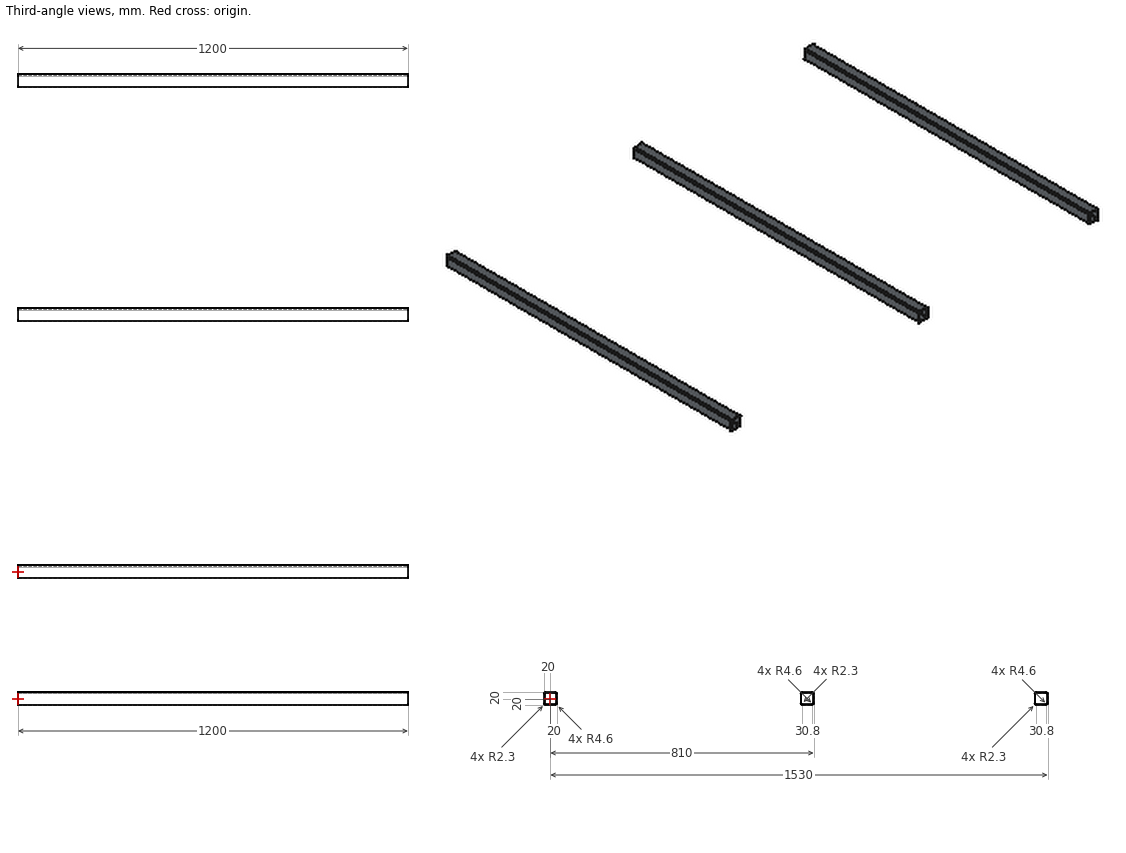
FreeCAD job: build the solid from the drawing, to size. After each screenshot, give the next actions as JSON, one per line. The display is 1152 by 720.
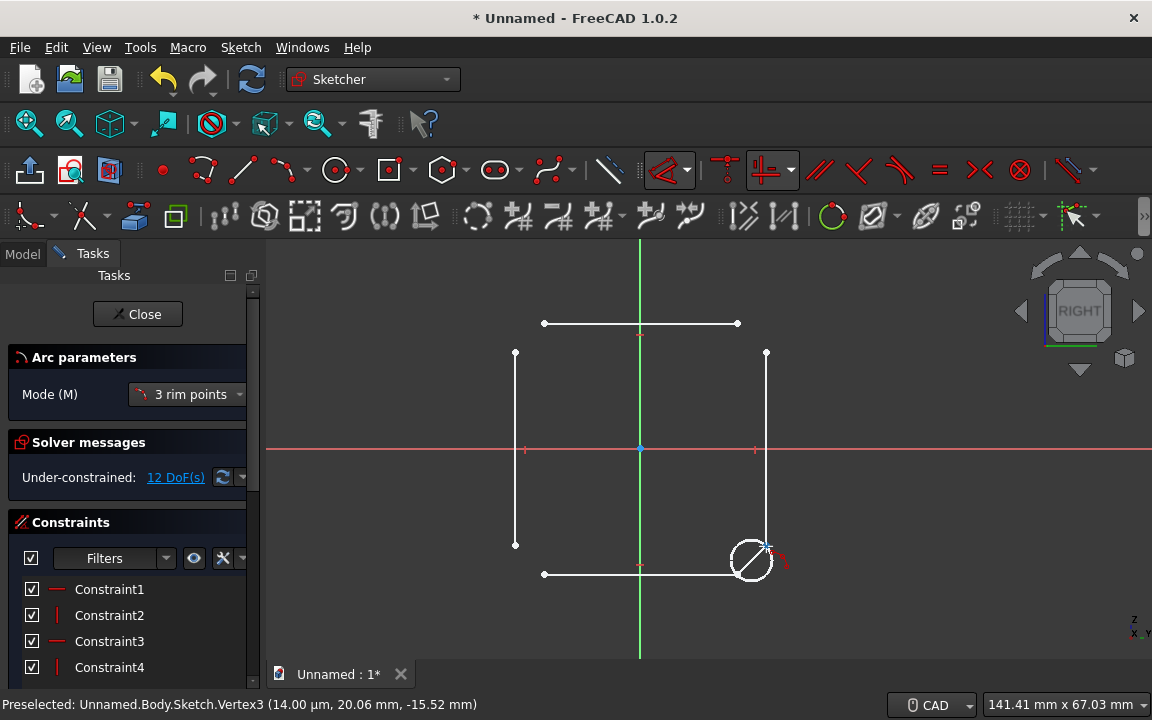
{"action": "scroll", "coordinate": [757, 566], "scroll_direction": "up", "scroll_amount": 4}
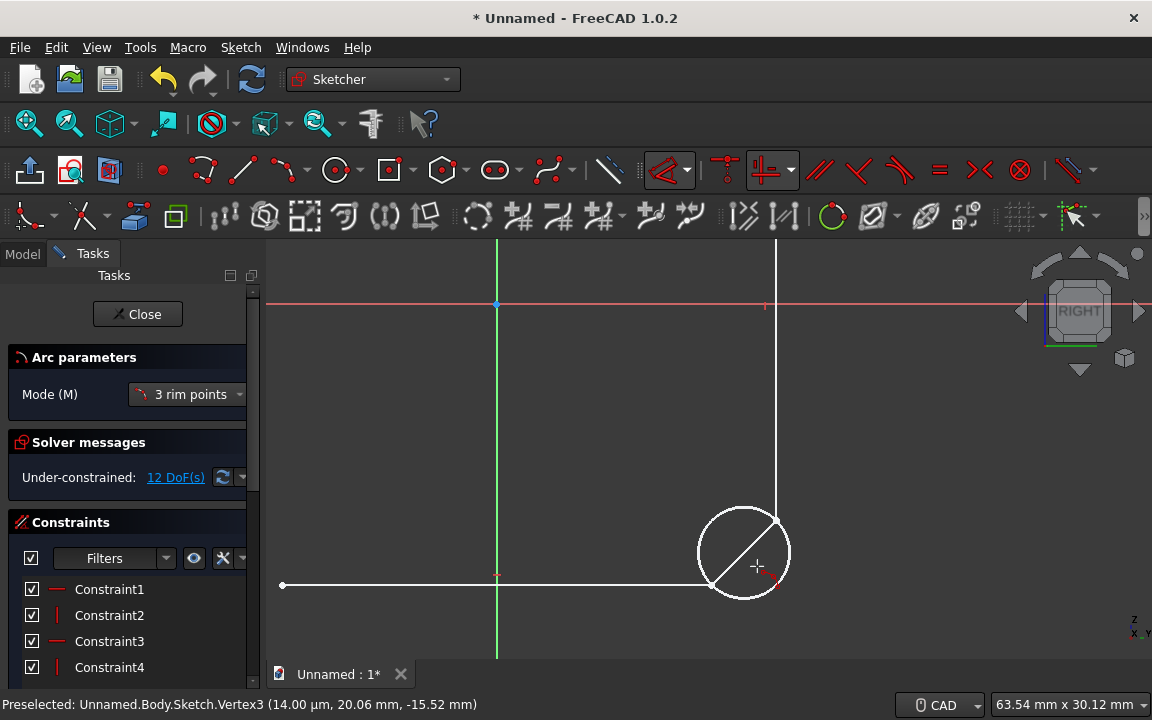
{"action": "left_click", "coordinate": [757, 564]}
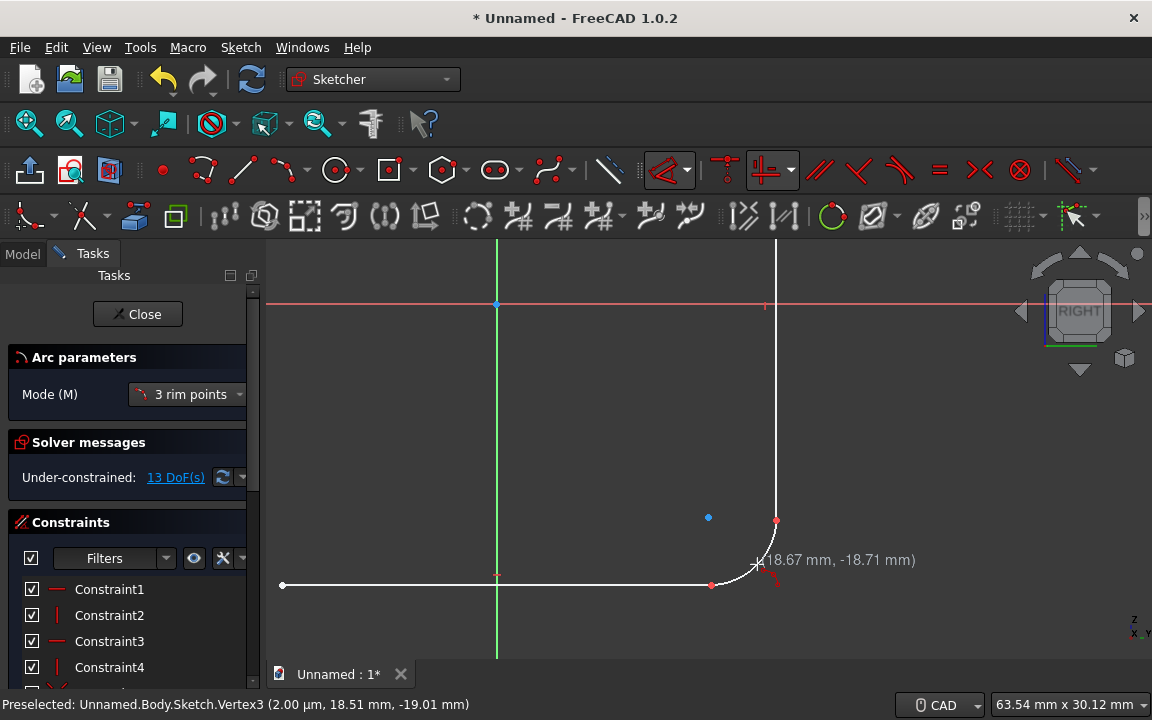
{"action": "scroll", "coordinate": [758, 567], "scroll_direction": "down", "scroll_amount": 4}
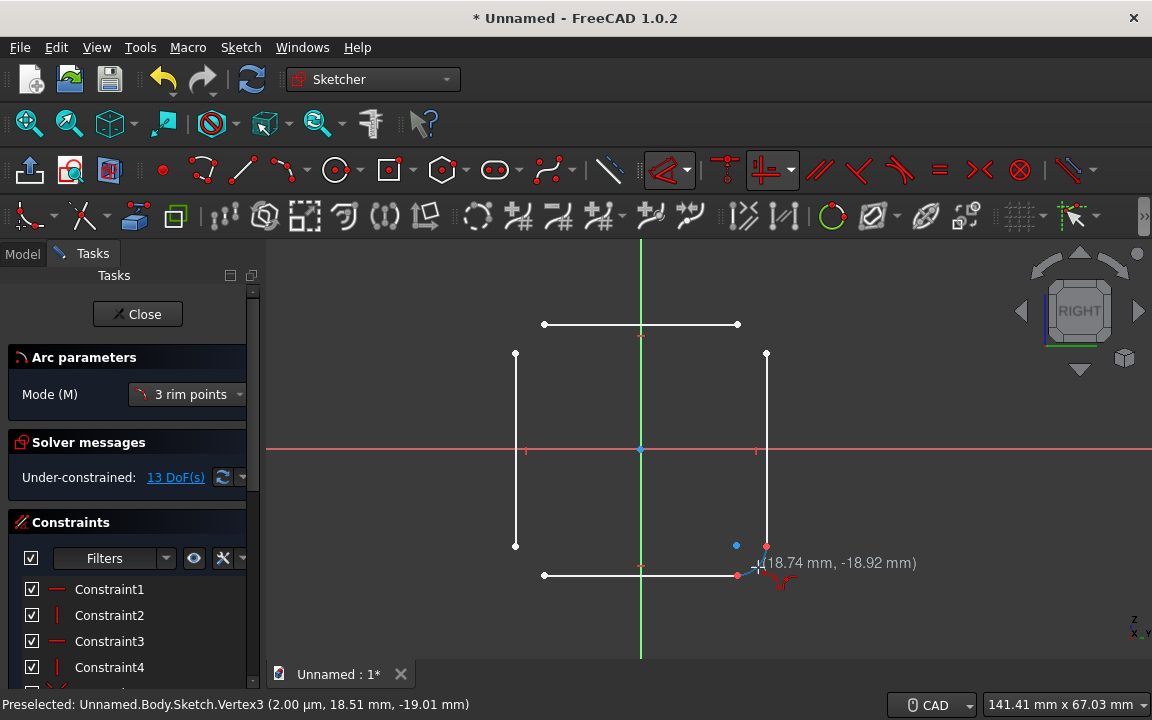
{"action": "left_click", "coordinate": [767, 354]}
{"action": "left_click", "coordinate": [738, 325]}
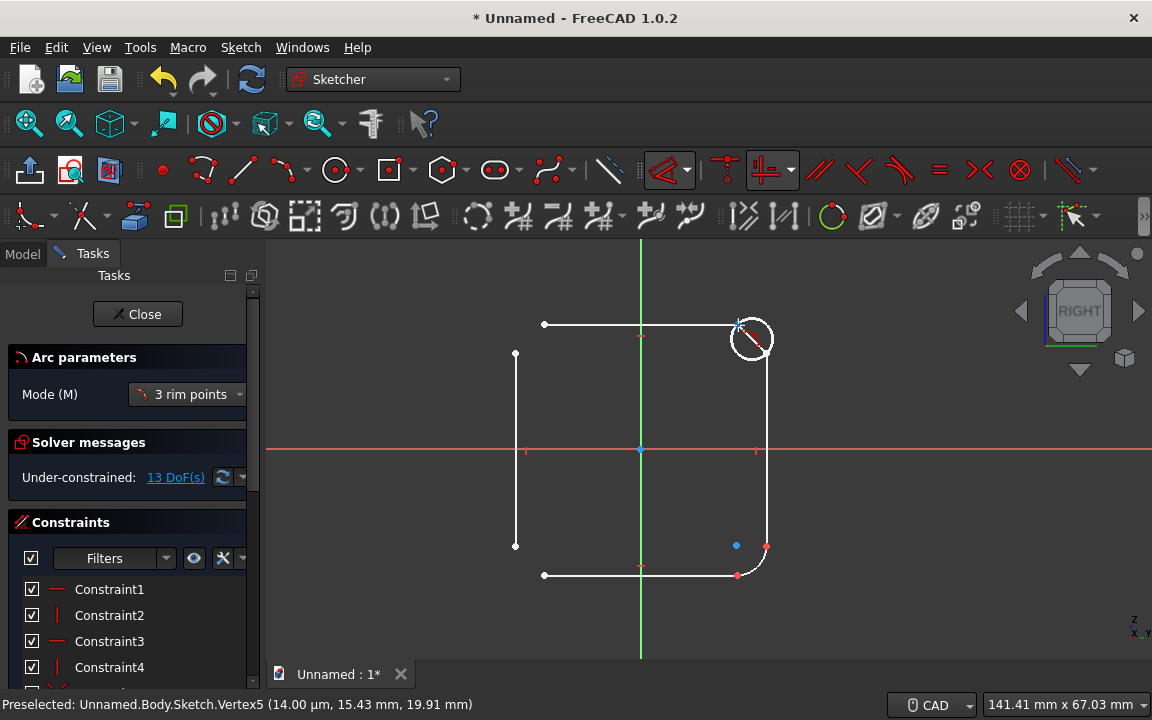
{"action": "scroll", "coordinate": [758, 332], "scroll_direction": "up", "scroll_amount": 4}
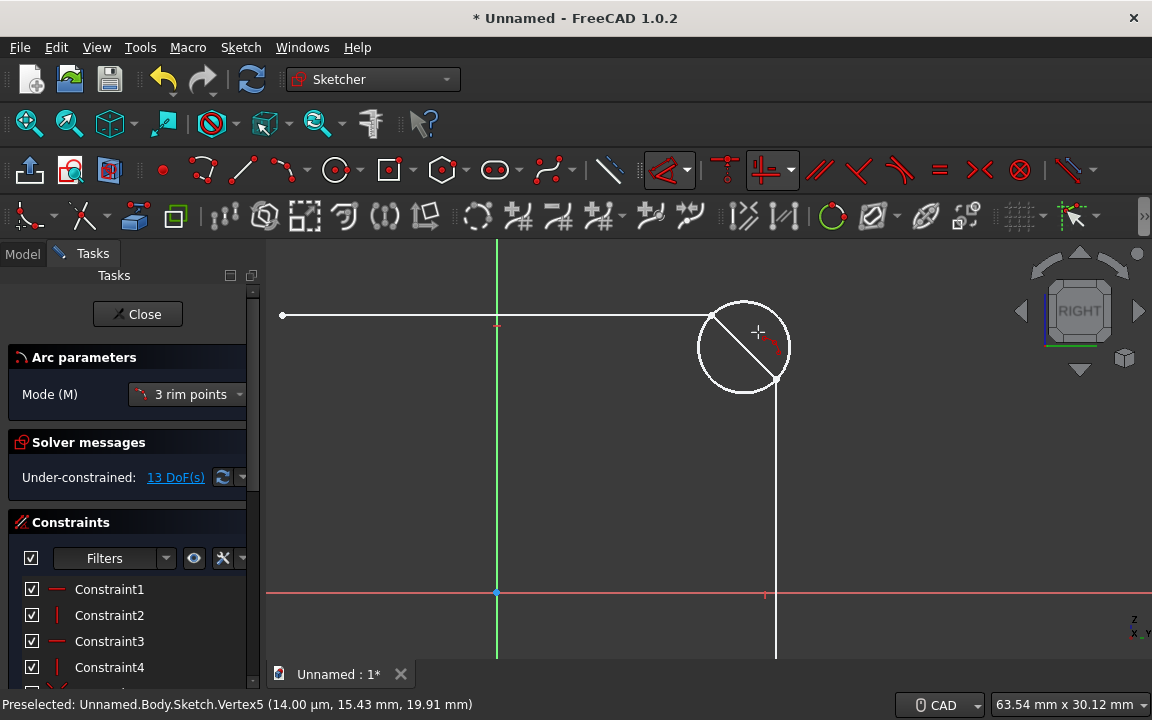
{"action": "left_click", "coordinate": [757, 333]}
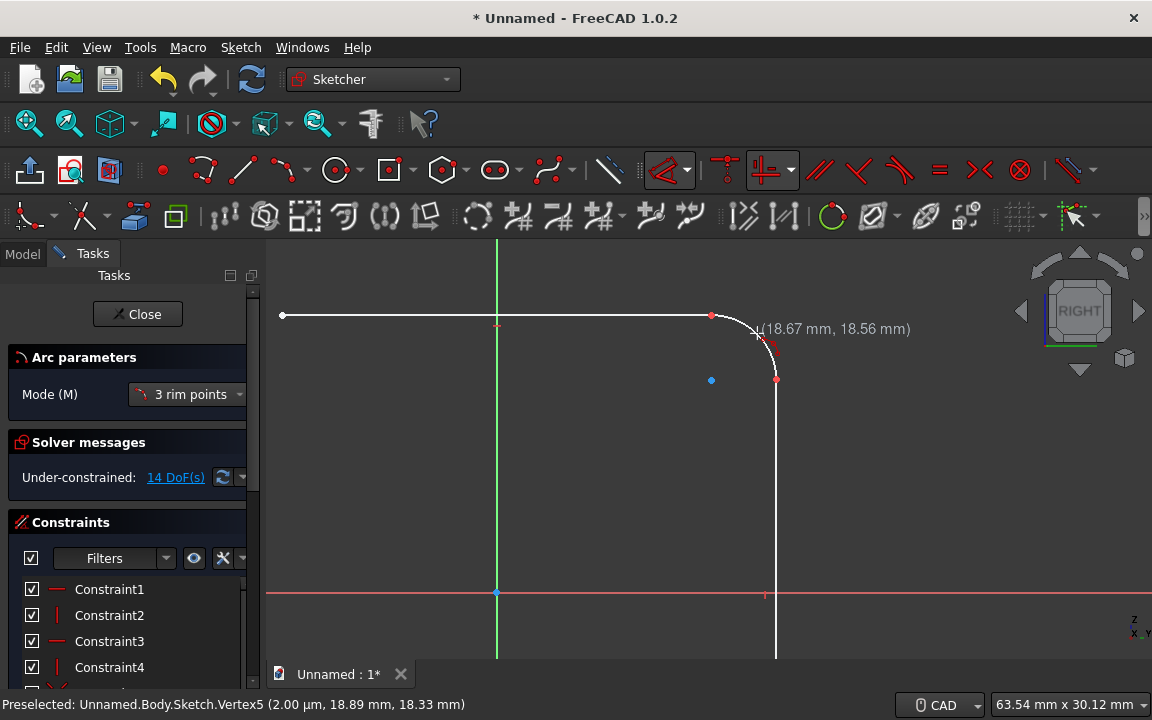
{"action": "scroll", "coordinate": [758, 332], "scroll_direction": "down", "scroll_amount": 4}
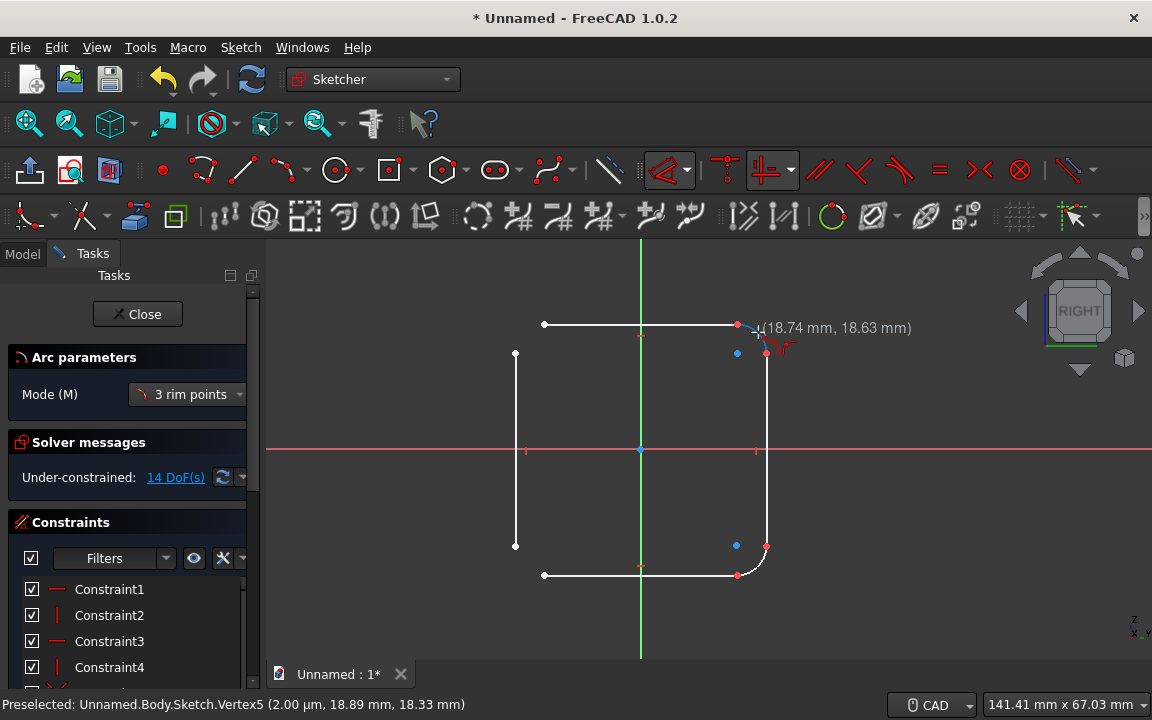
{"action": "left_click", "coordinate": [545, 325]}
{"action": "left_click", "coordinate": [516, 354]}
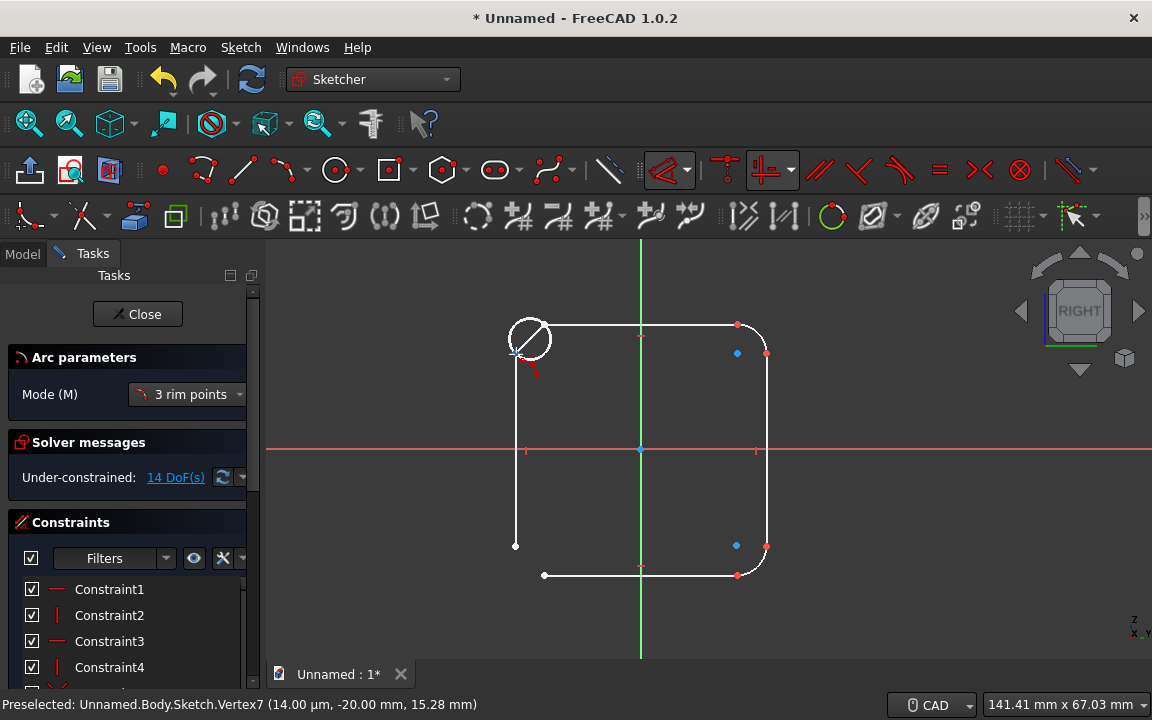
{"action": "scroll", "coordinate": [524, 332], "scroll_direction": "up", "scroll_amount": 4}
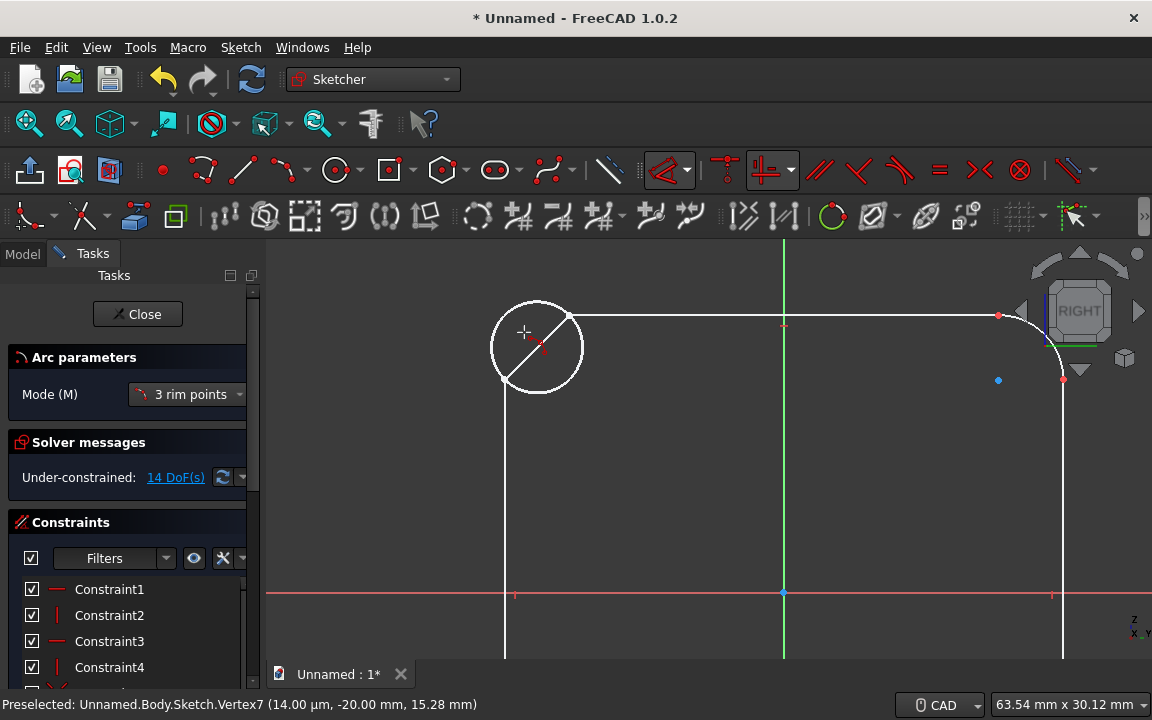
{"action": "left_click", "coordinate": [524, 333]}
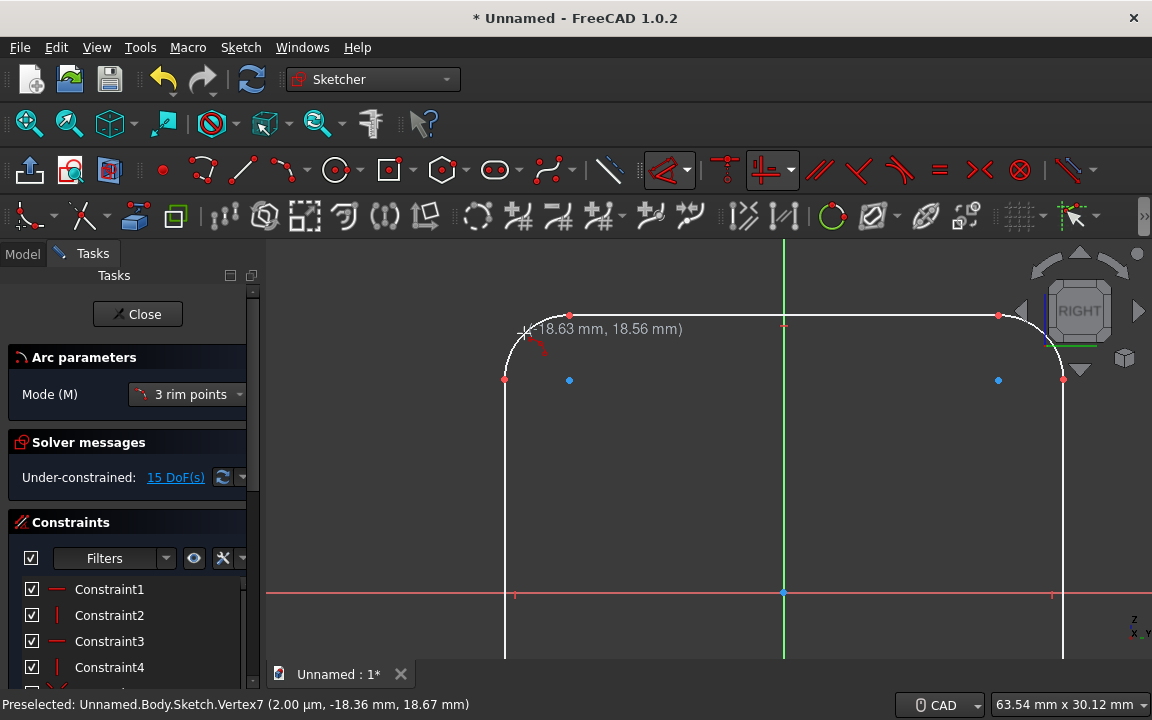
{"action": "scroll", "coordinate": [524, 332], "scroll_direction": "down", "scroll_amount": 4}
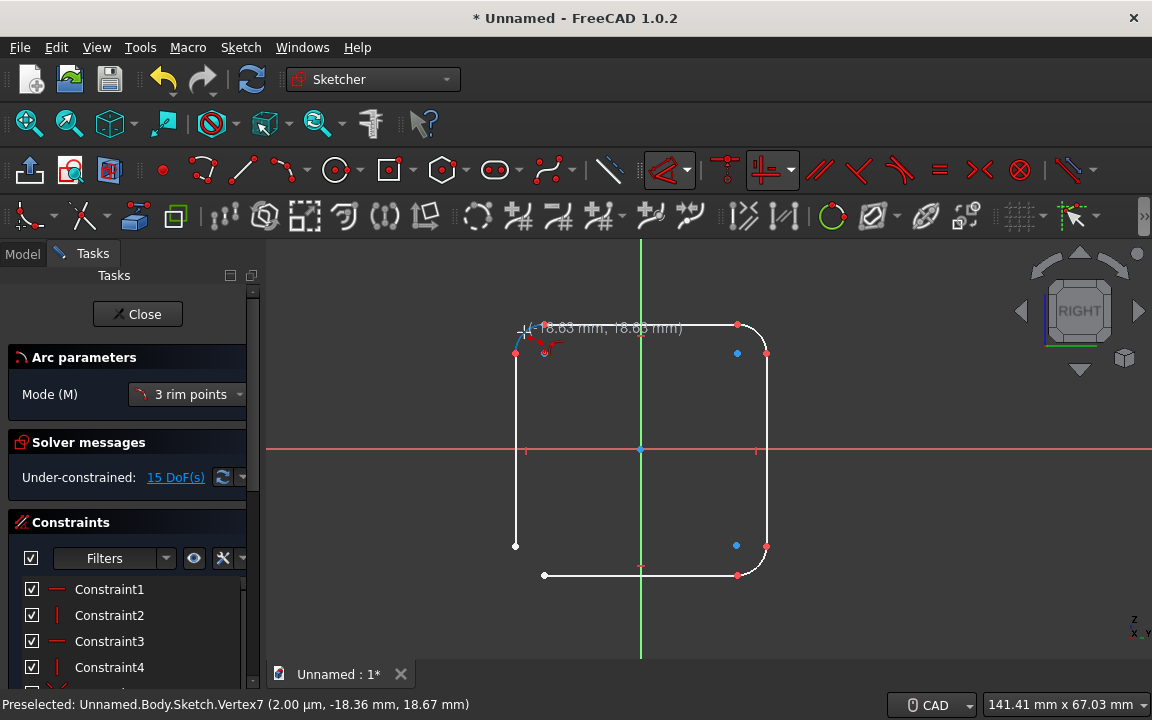
{"action": "left_click", "coordinate": [516, 547]}
{"action": "left_click", "coordinate": [545, 576]}